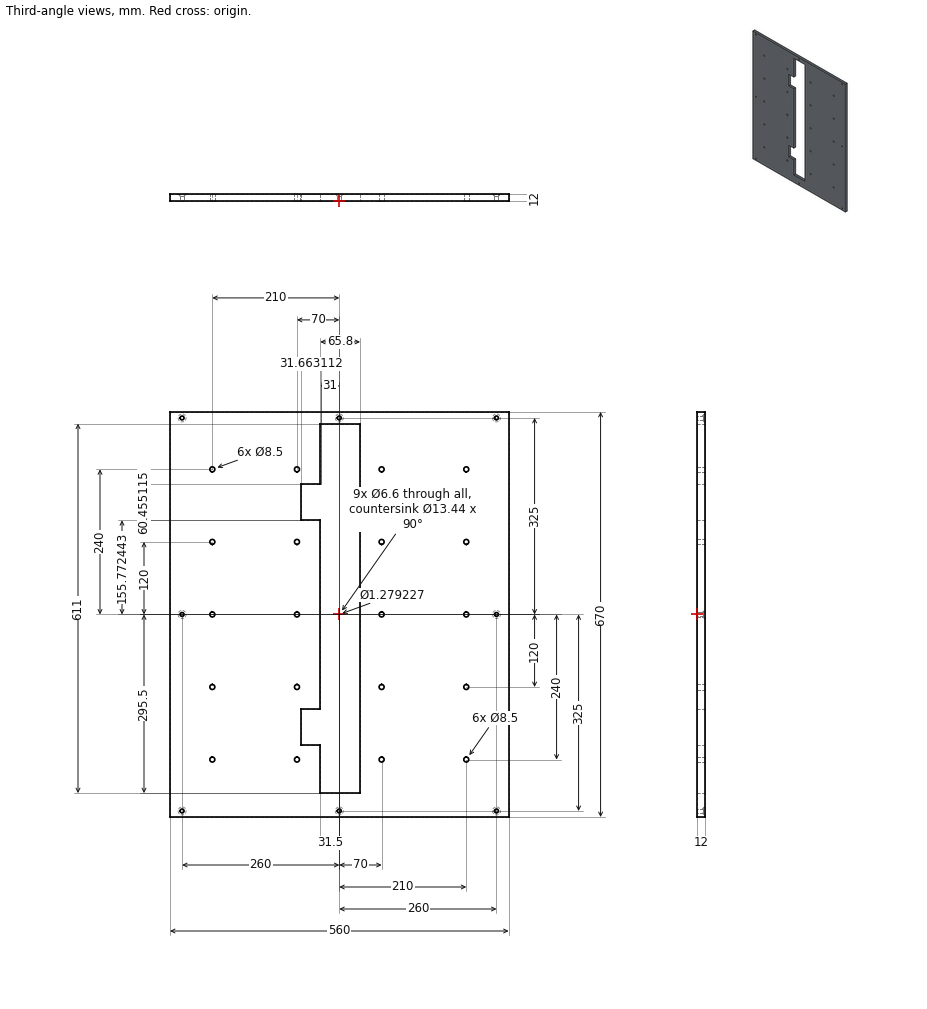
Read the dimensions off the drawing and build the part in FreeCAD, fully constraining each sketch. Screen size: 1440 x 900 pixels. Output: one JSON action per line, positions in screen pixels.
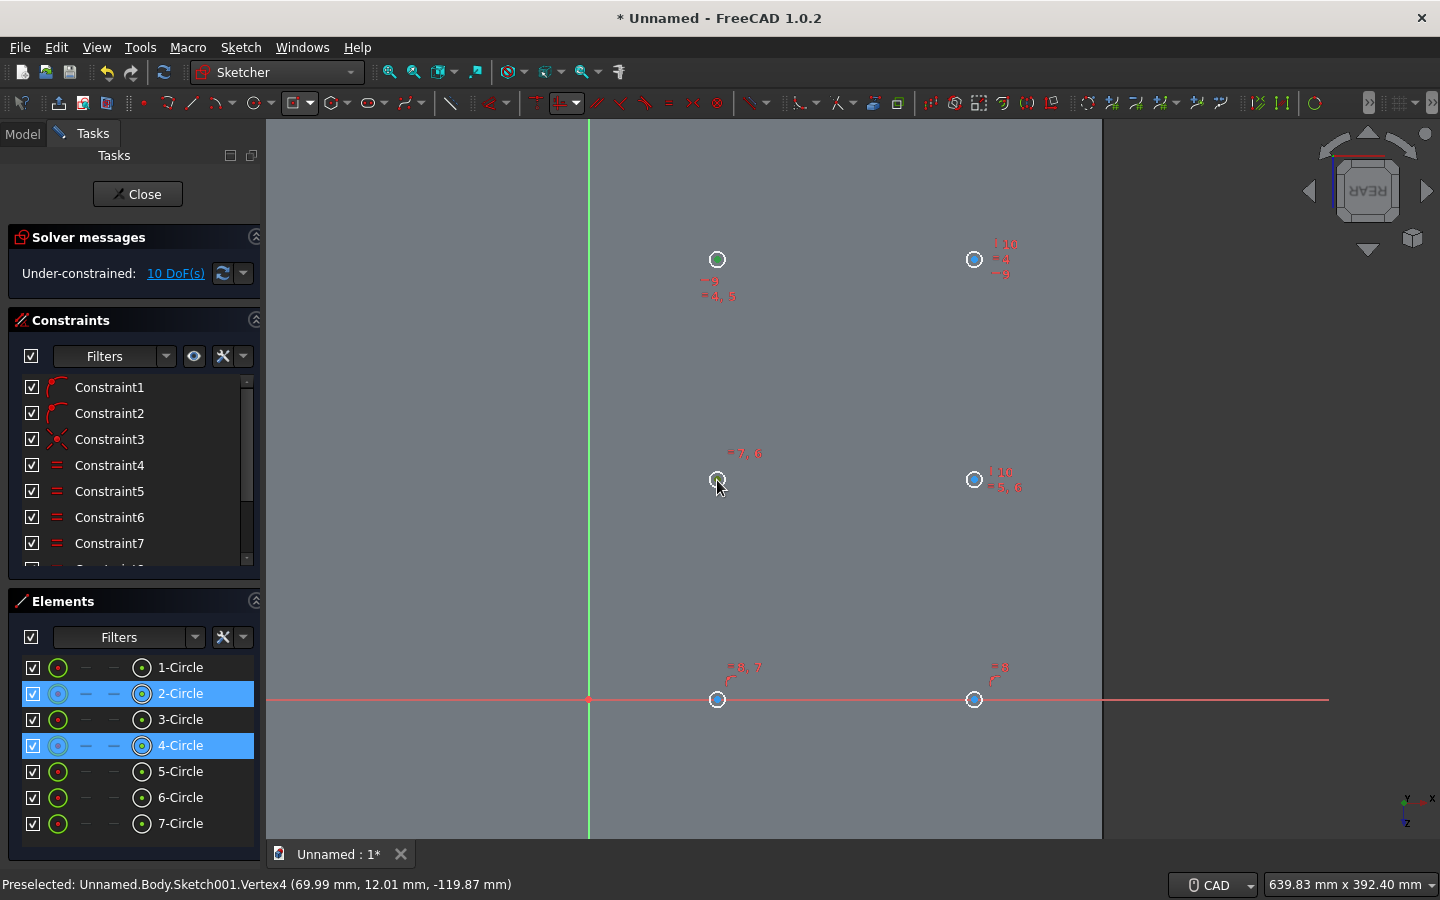
{"action": "key", "text": "v"}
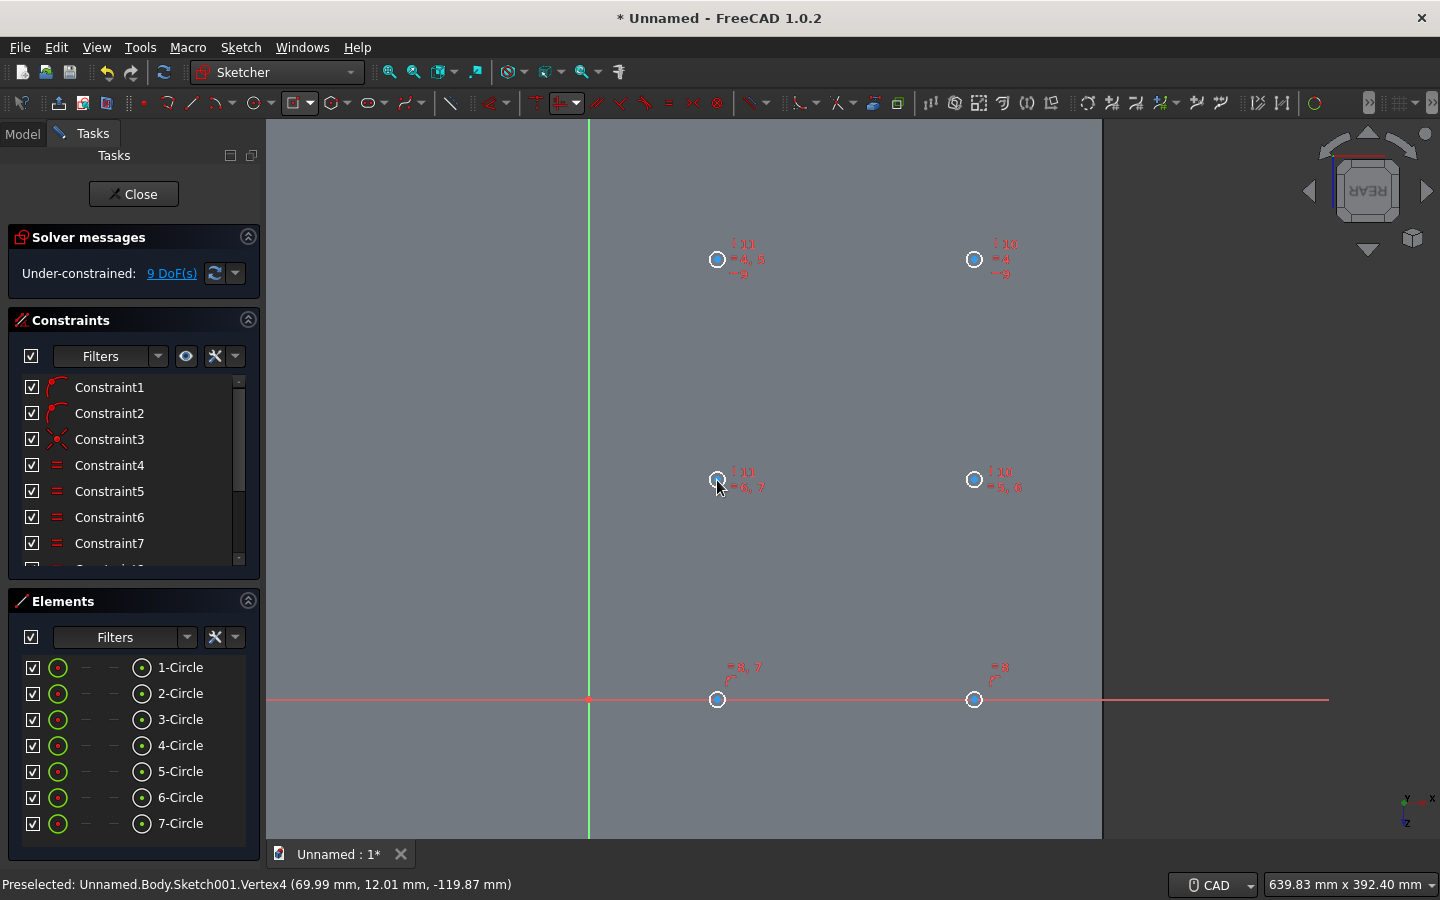
{"action": "left_click", "coordinate": [974, 480]}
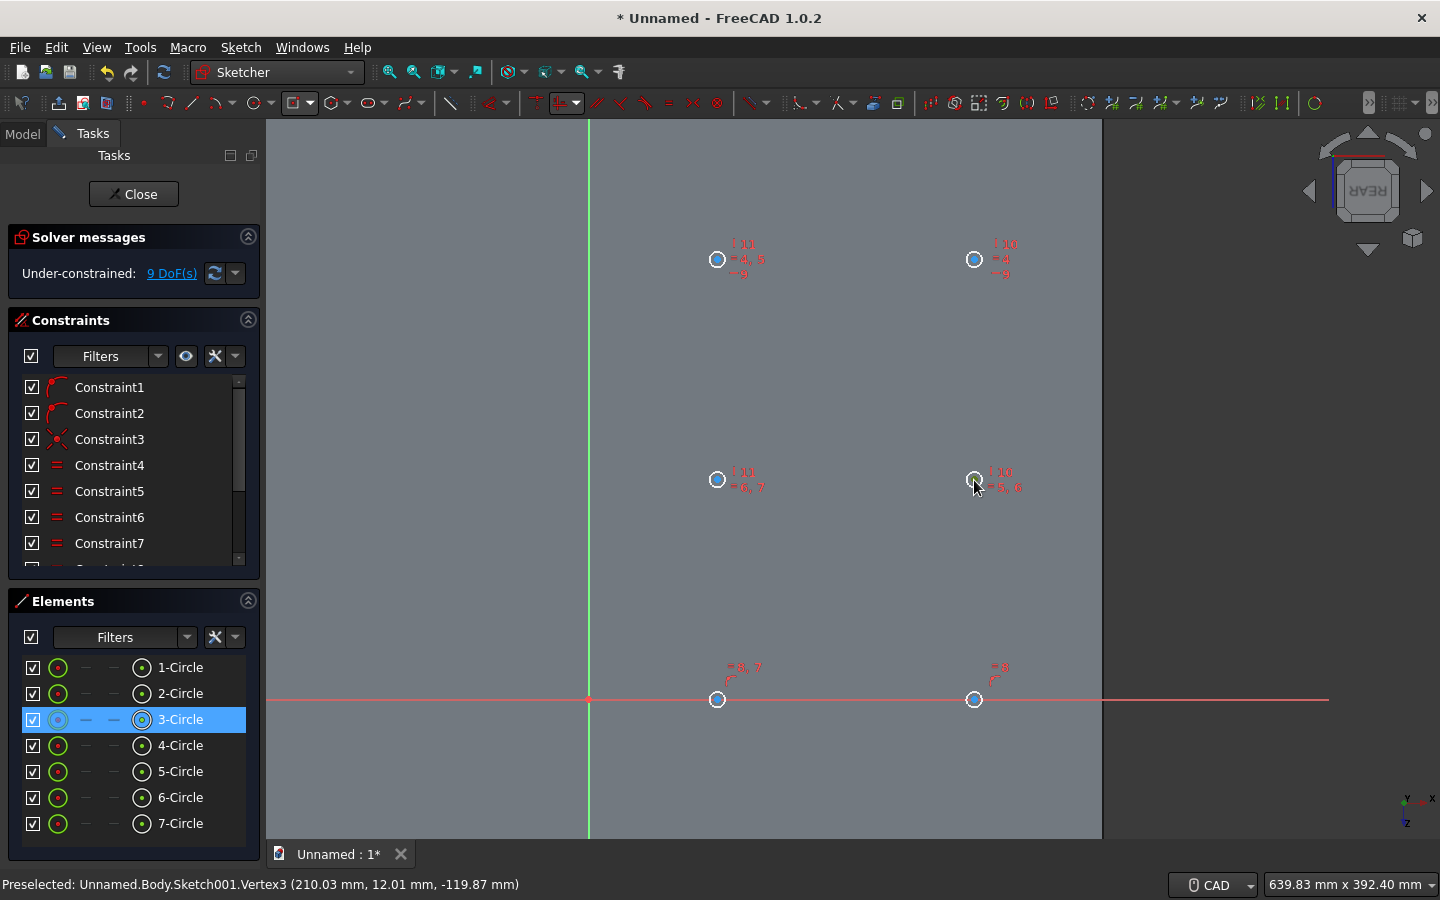
{"action": "left_click", "coordinate": [717, 480]}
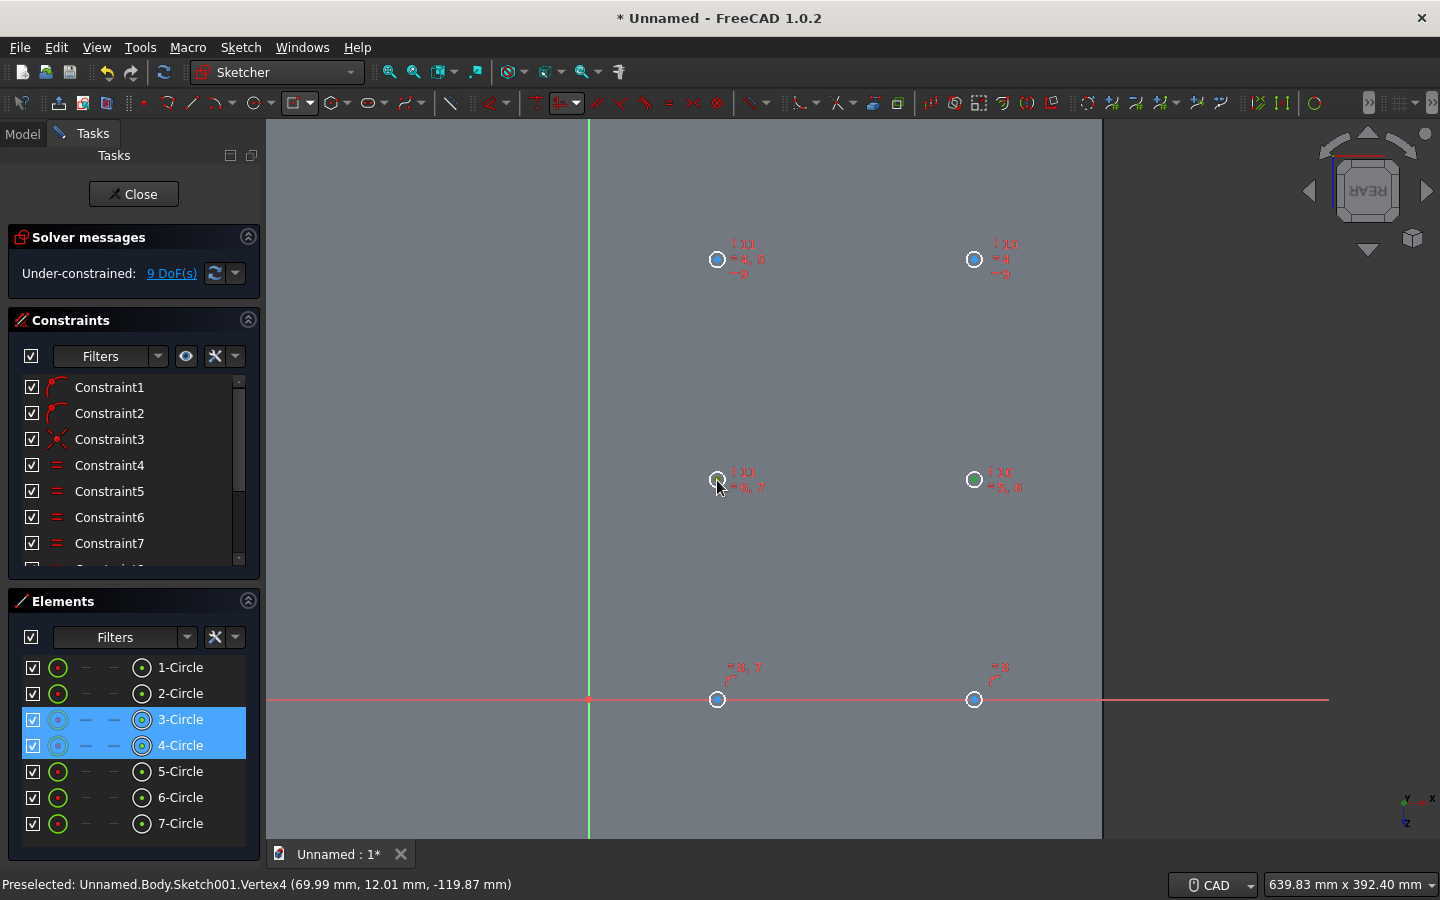
{"action": "left_click", "coordinate": [578, 104]}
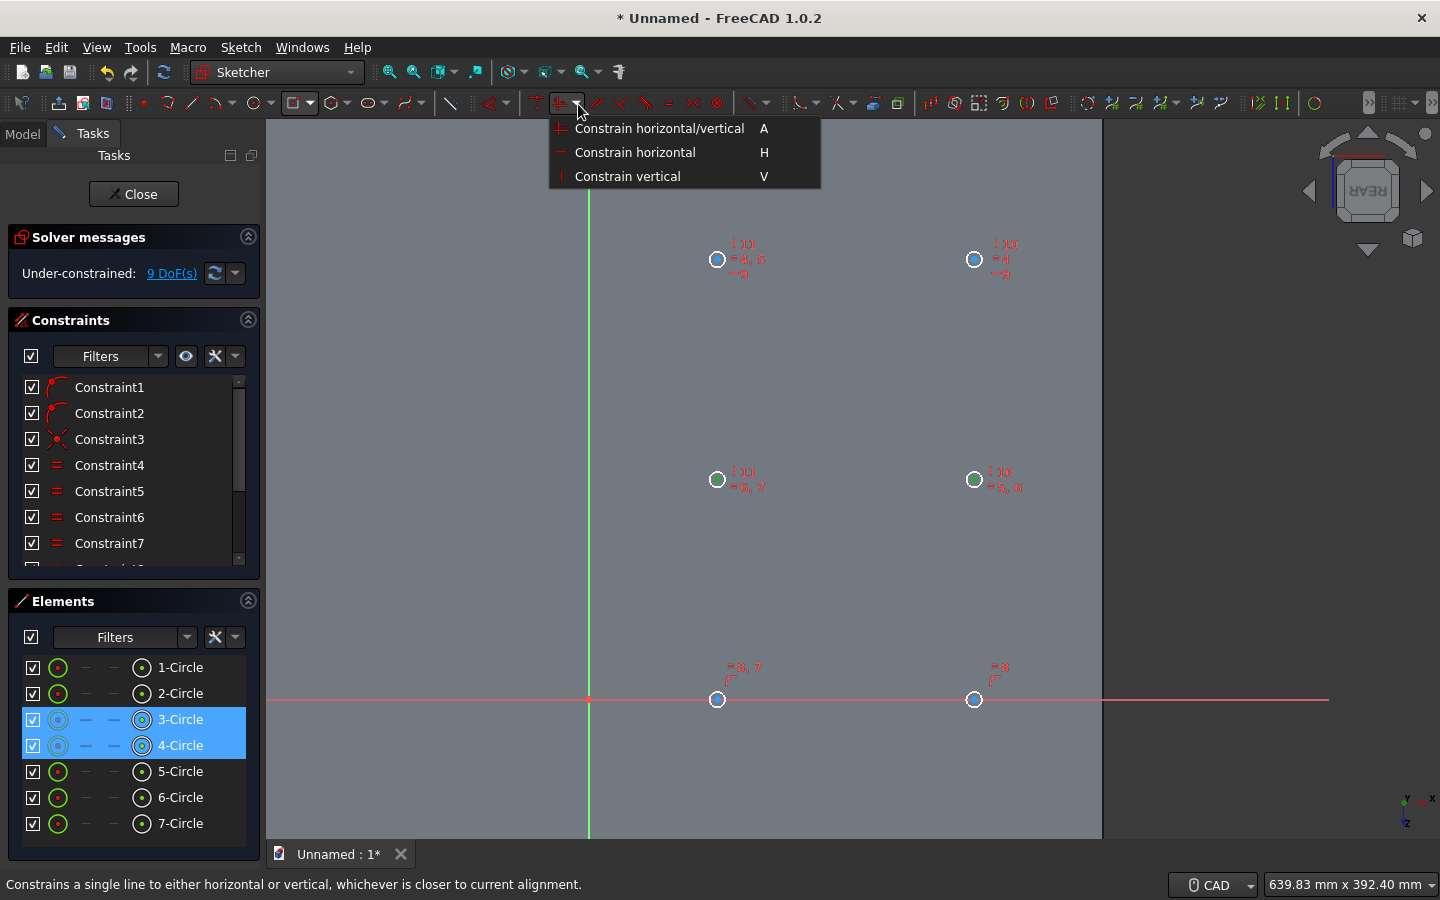
{"action": "left_click", "coordinate": [685, 152]}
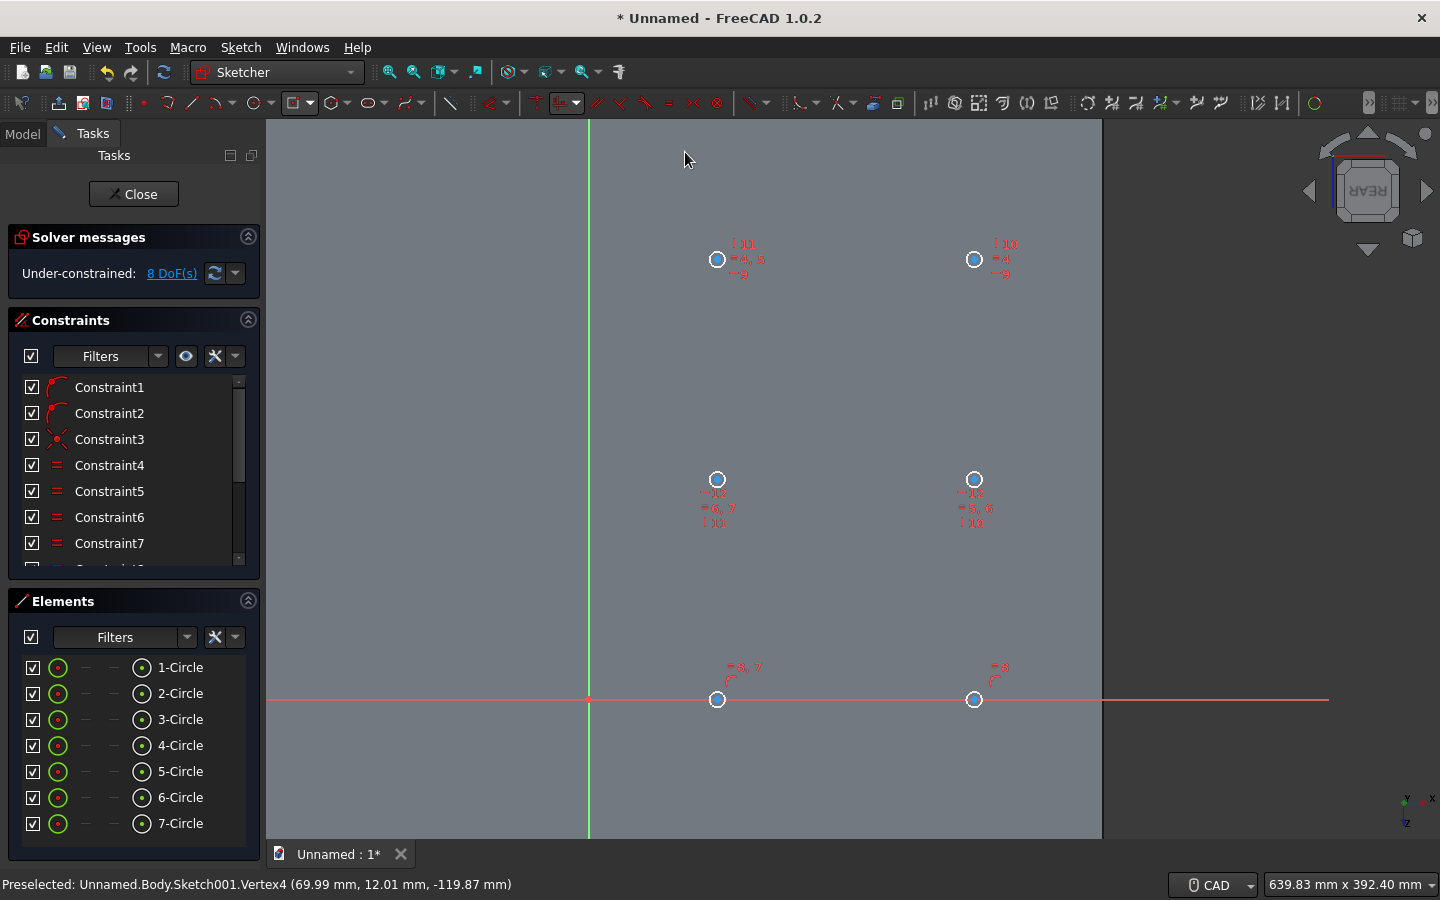
{"action": "left_click", "coordinate": [717, 480]}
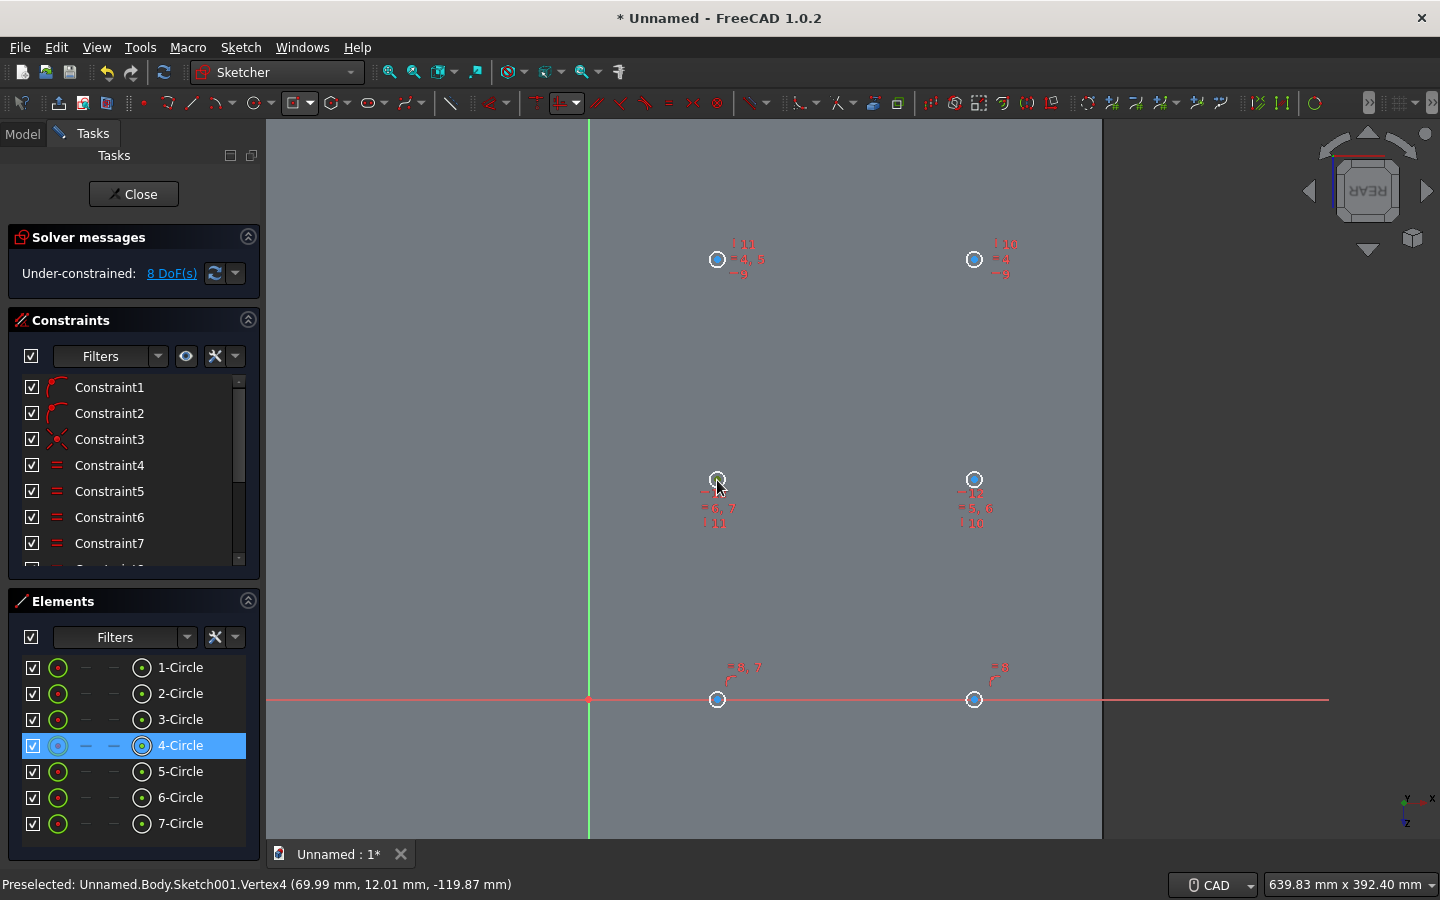
{"action": "left_click", "coordinate": [717, 700]}